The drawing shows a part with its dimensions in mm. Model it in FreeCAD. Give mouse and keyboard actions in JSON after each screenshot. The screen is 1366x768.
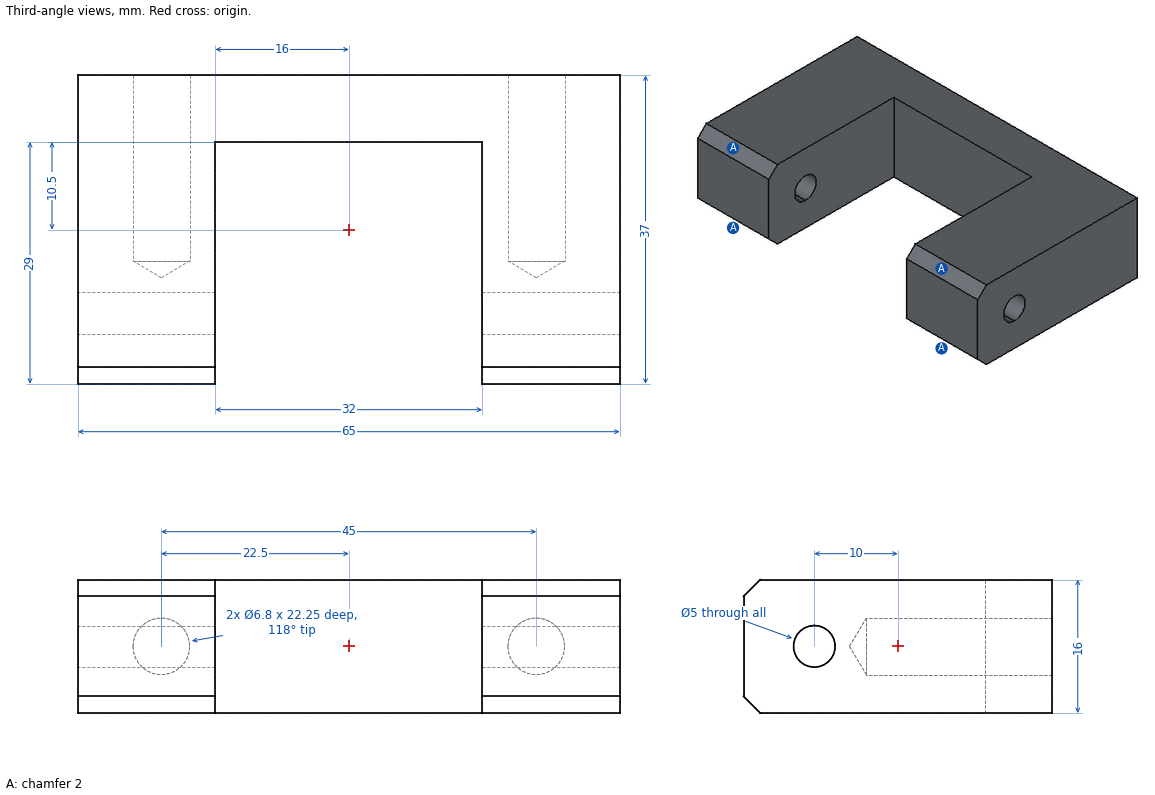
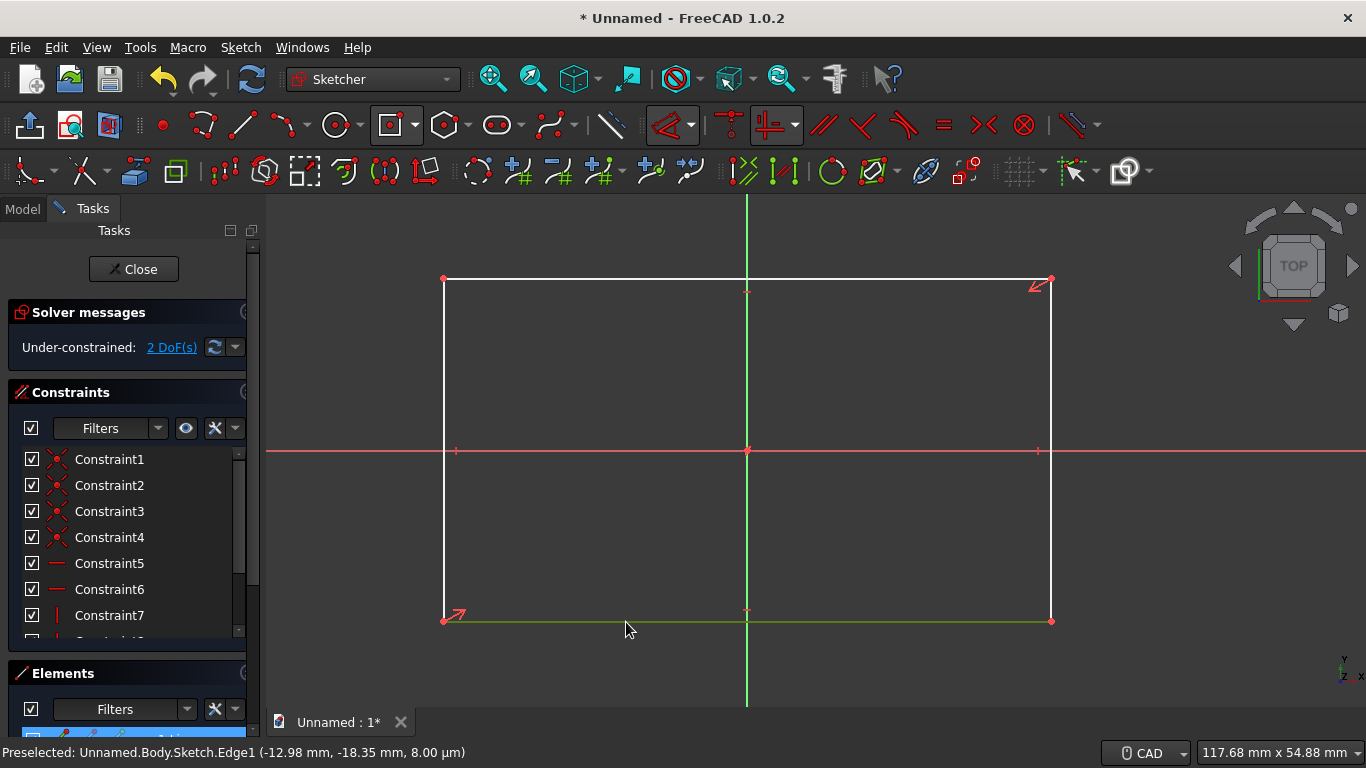
{"action": "key", "text": "l"}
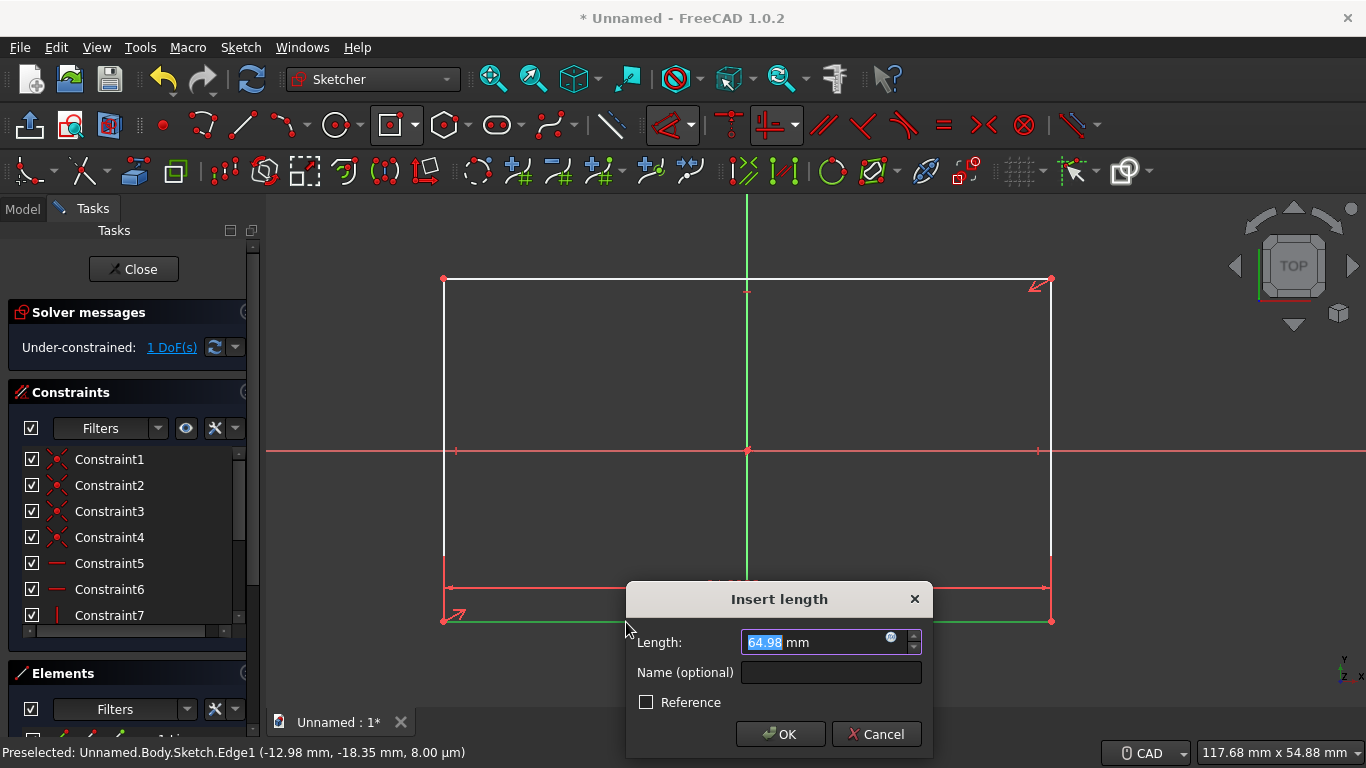
{"action": "type", "text": "65"}
{"action": "key", "text": "Return"}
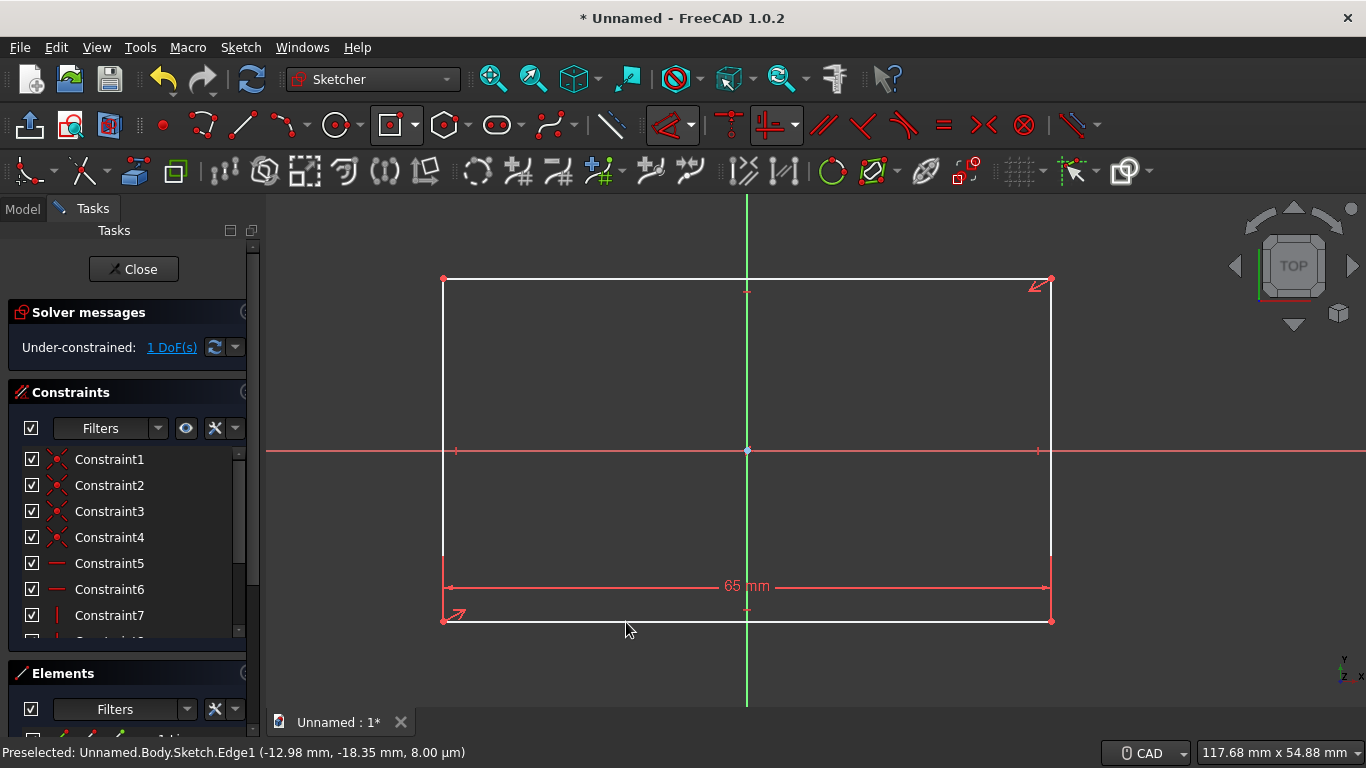
{"action": "left_click", "coordinate": [1051, 519]}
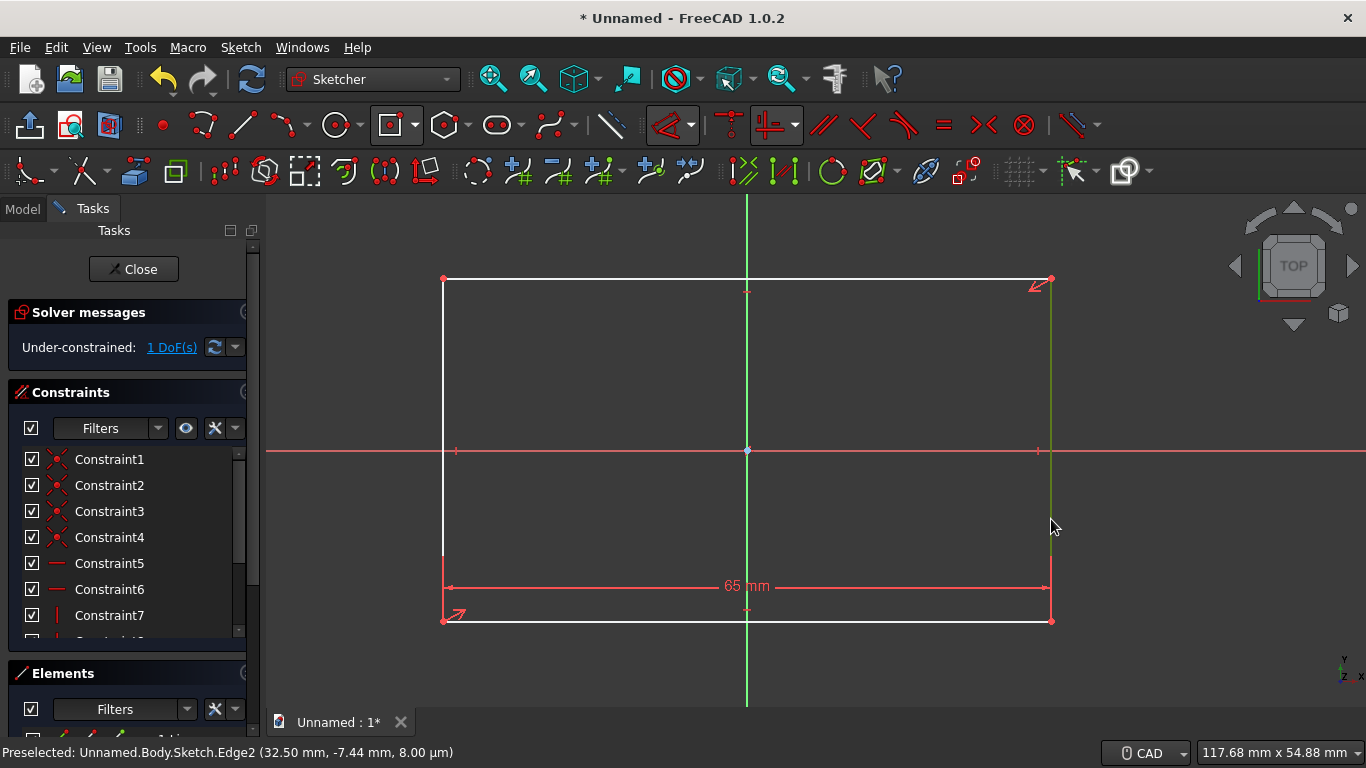
{"action": "left_click", "coordinate": [694, 126]}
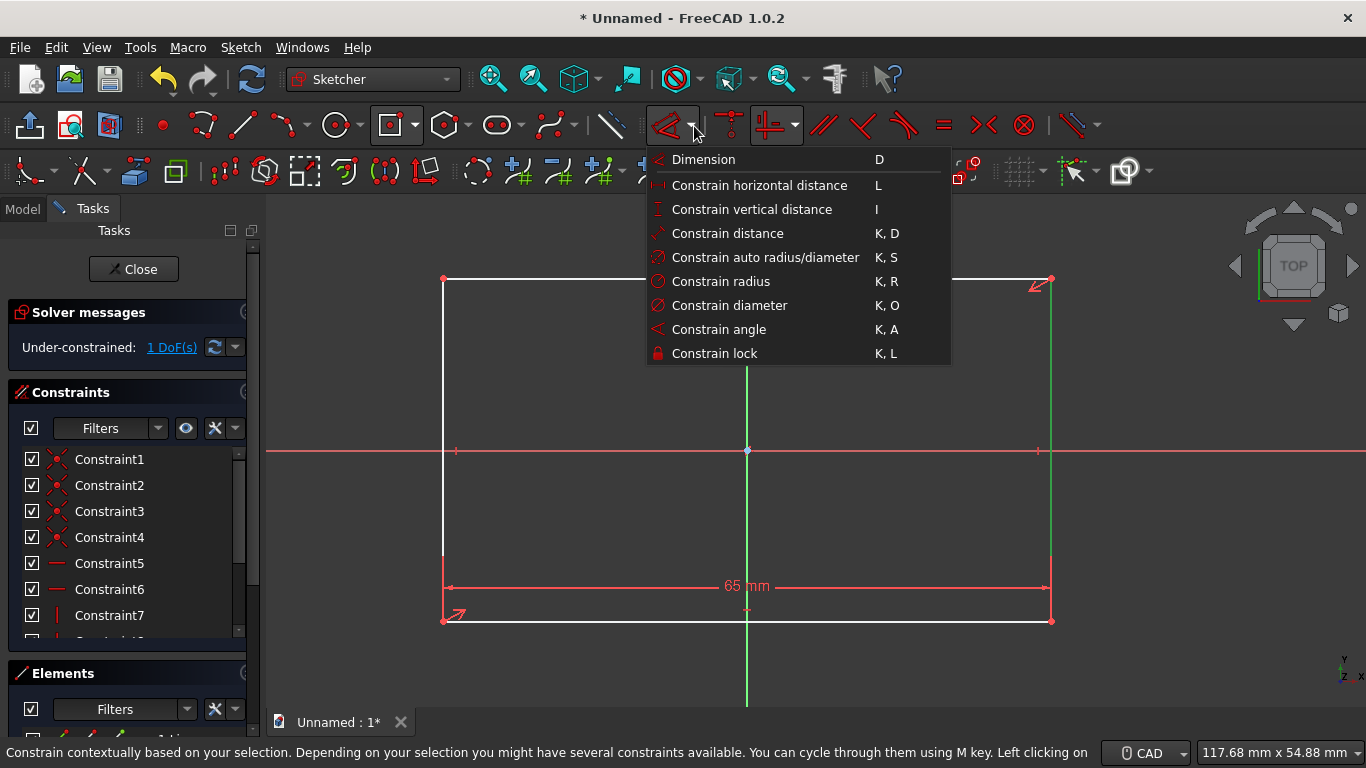
{"action": "left_click", "coordinate": [799, 209]}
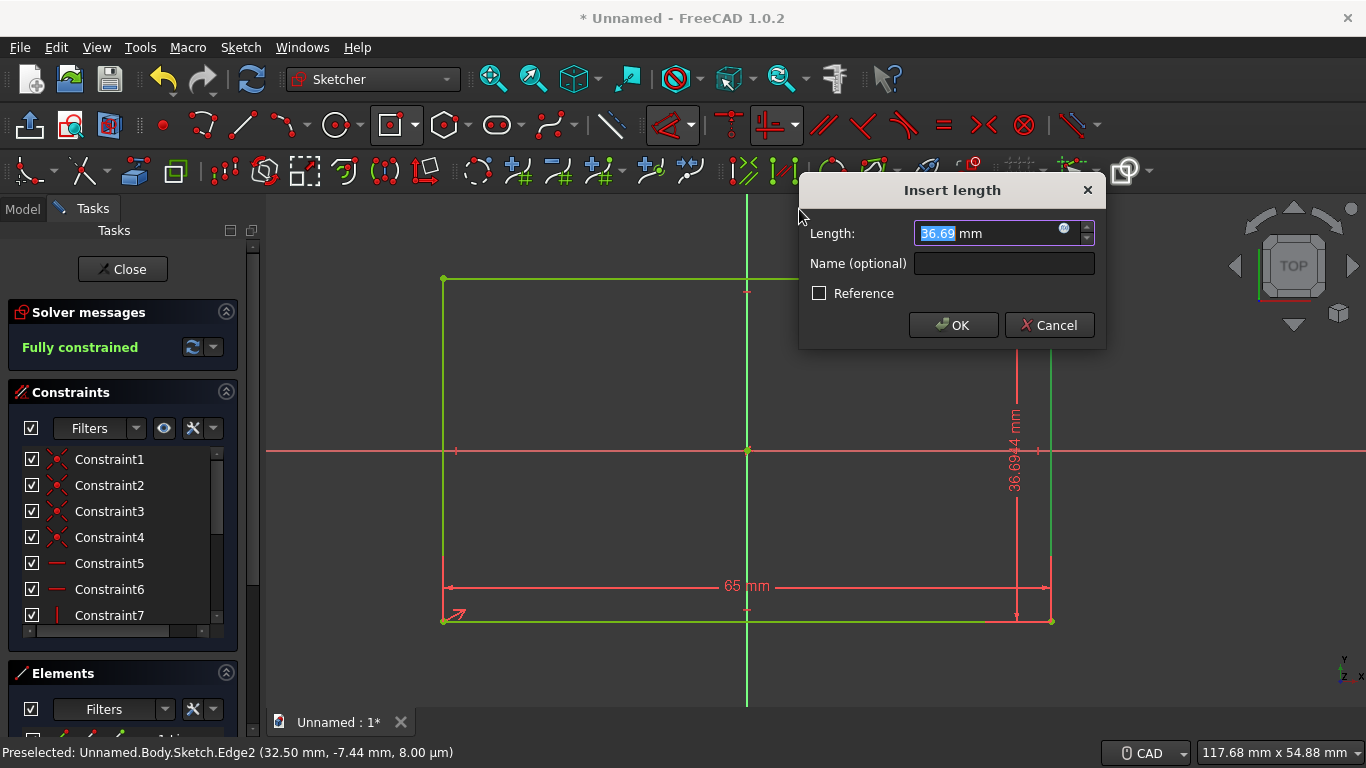
{"action": "type", "text": "37"}
{"action": "key", "text": "Return"}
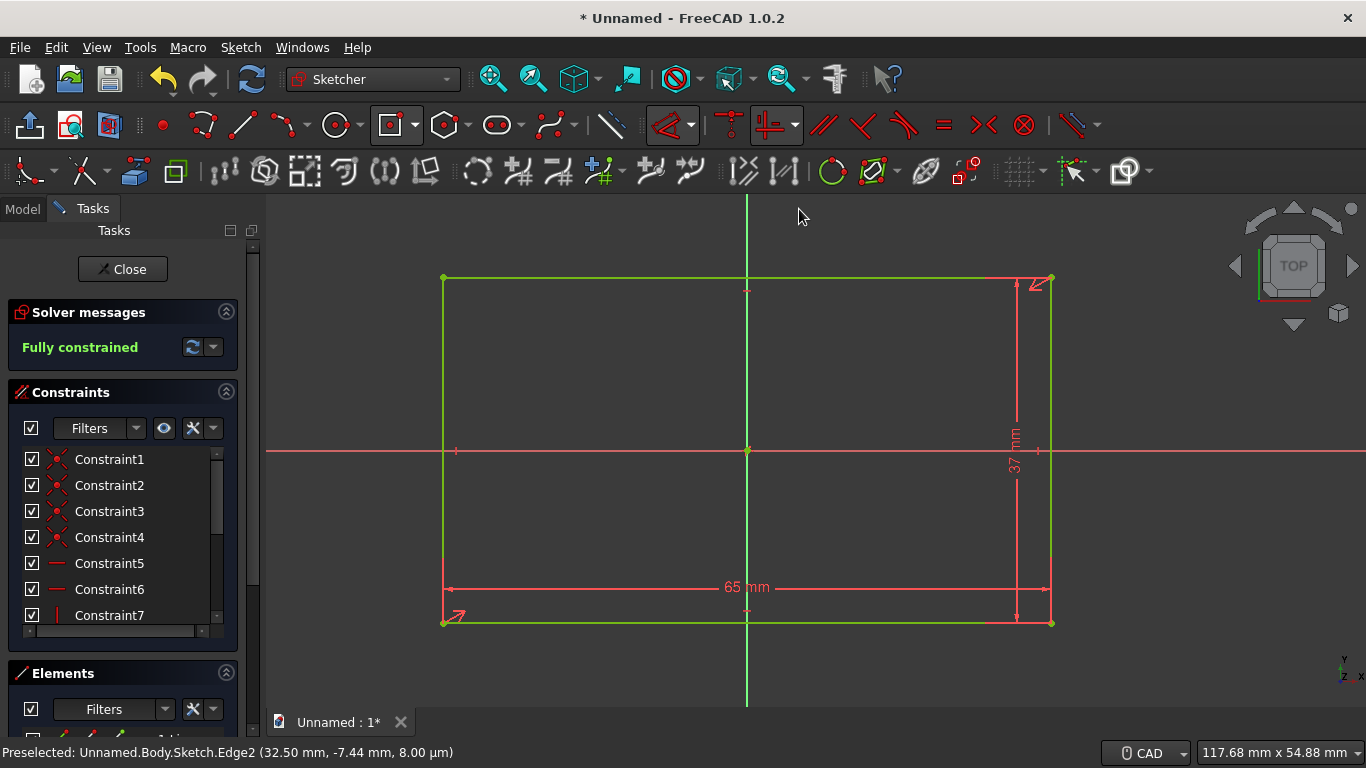
{"action": "left_click", "coordinate": [123, 269]}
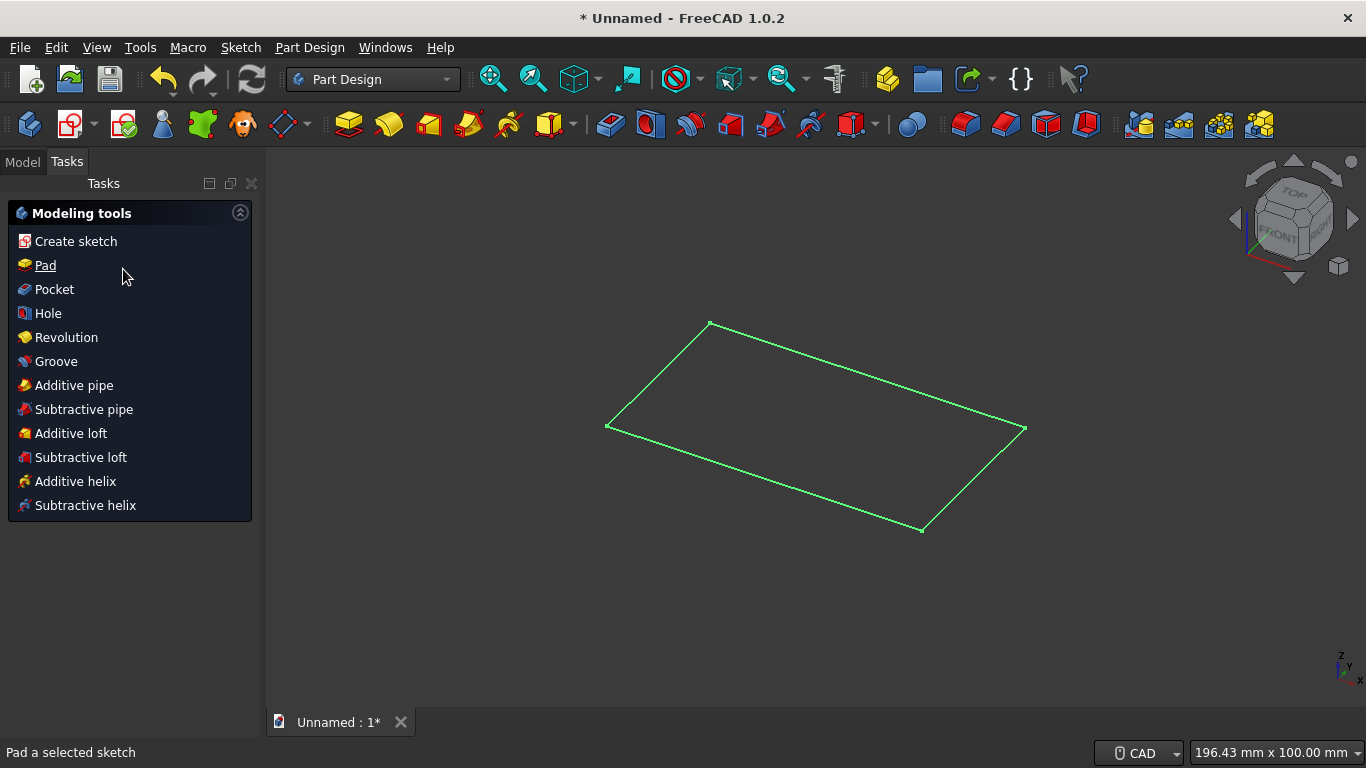
{"action": "left_click", "coordinate": [350, 124]}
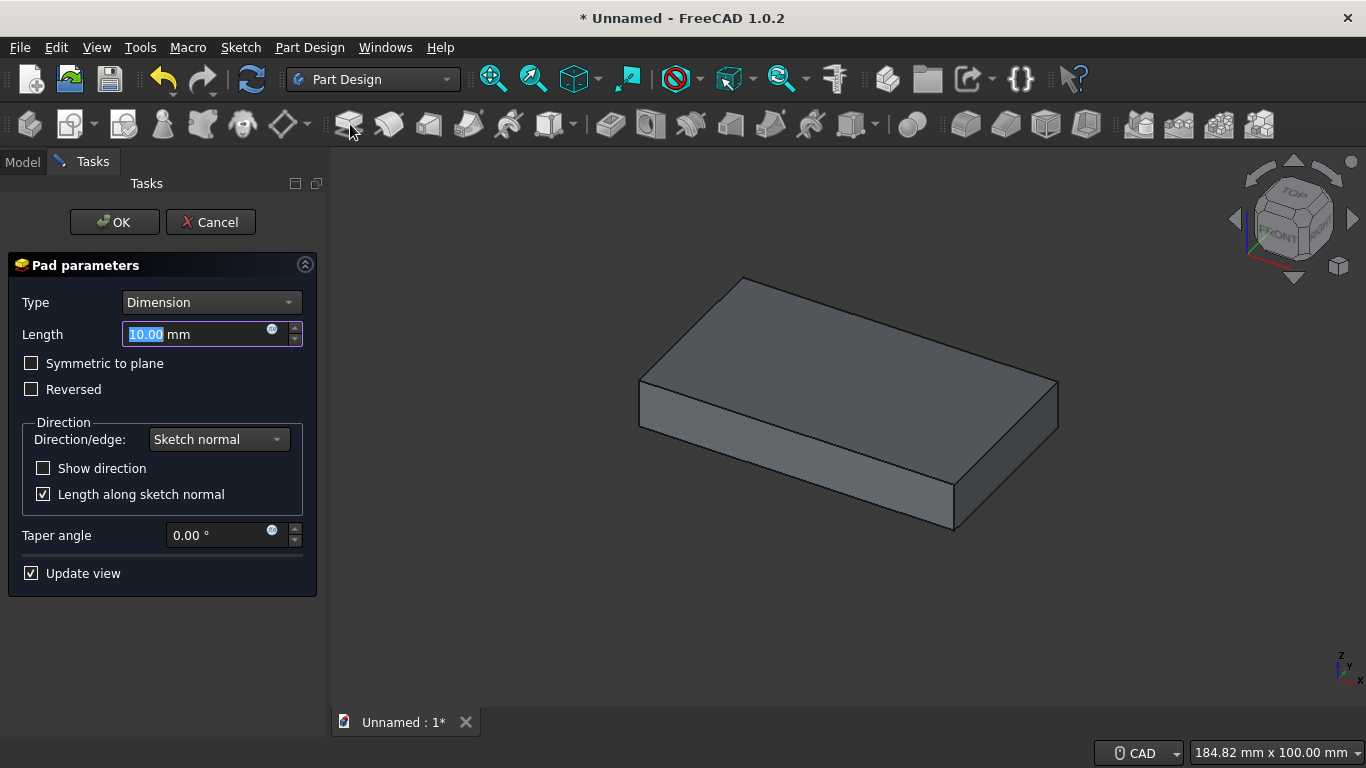
{"action": "type", "text": "16"}
{"action": "key", "text": "Tab"}